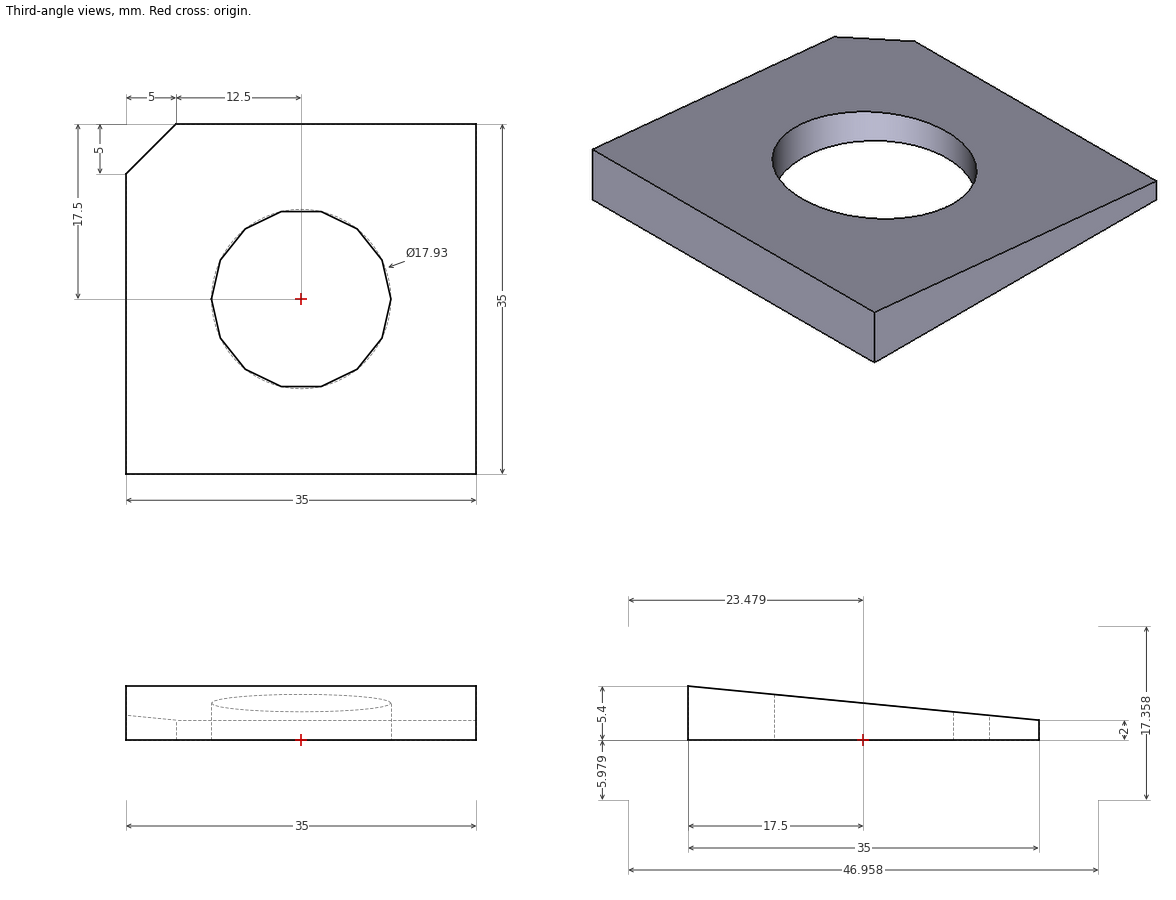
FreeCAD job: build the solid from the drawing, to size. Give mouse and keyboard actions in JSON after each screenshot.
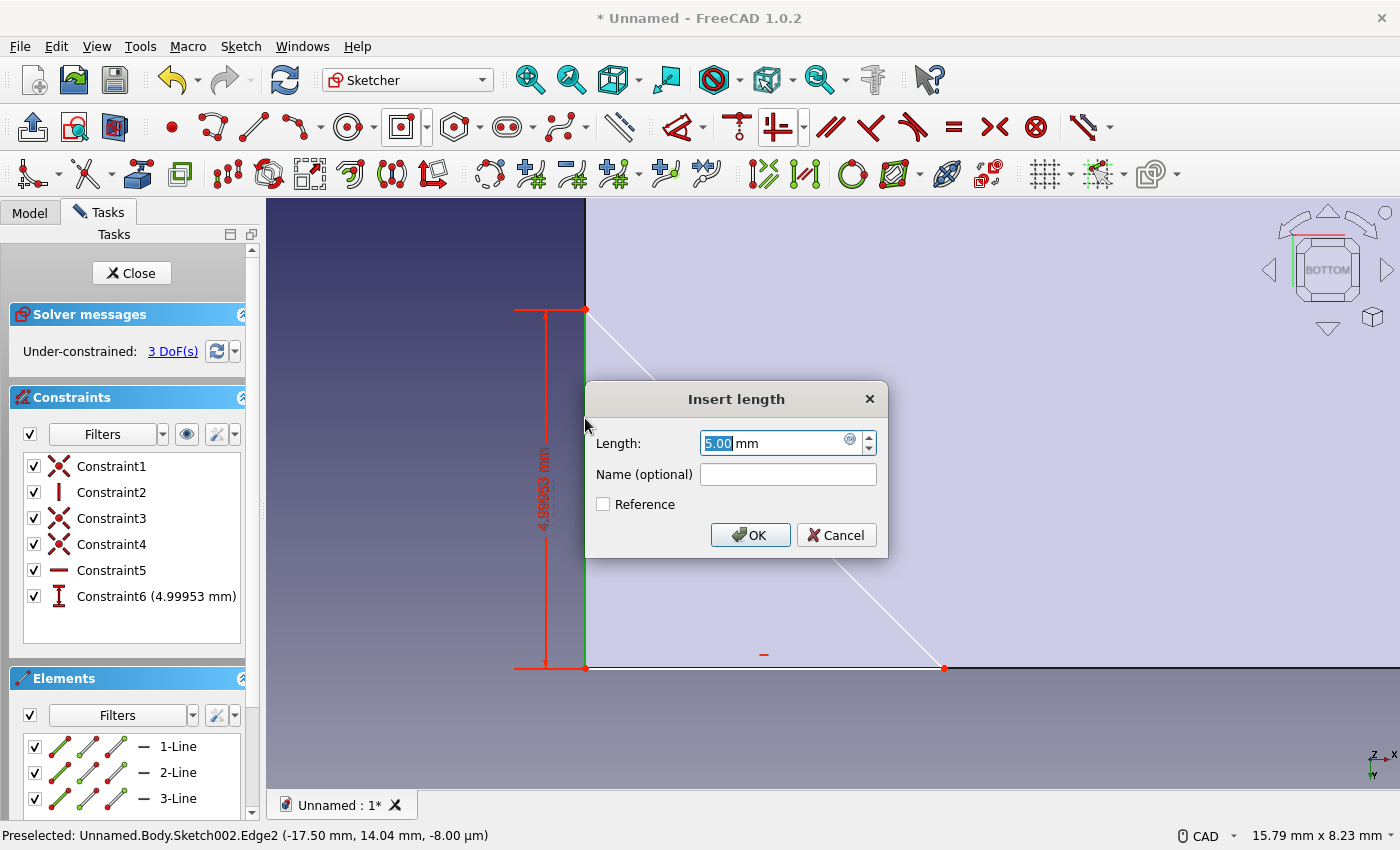
{"action": "type", "text": "5"}
{"action": "key", "text": "Return"}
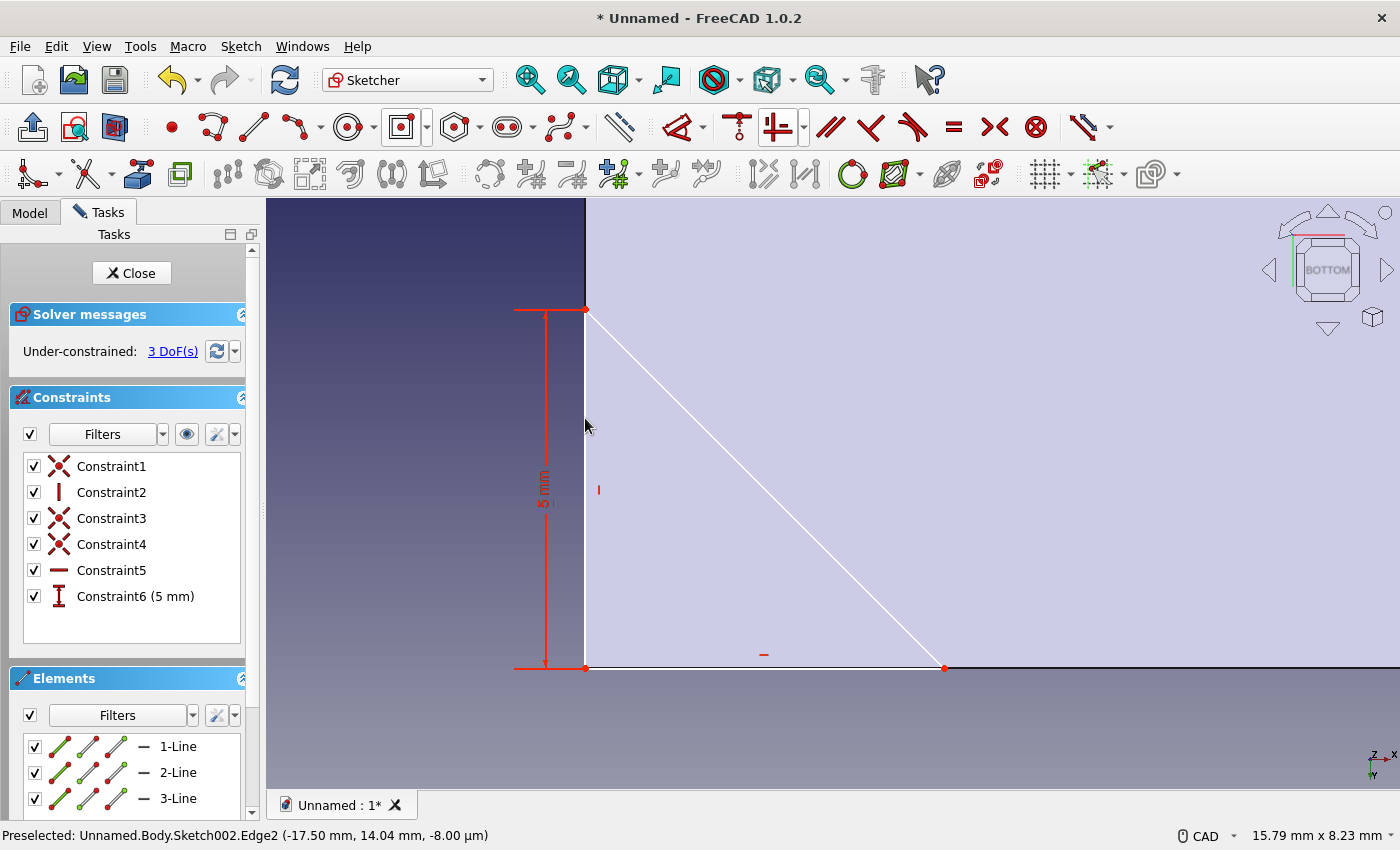
{"action": "left_click", "coordinate": [693, 669]}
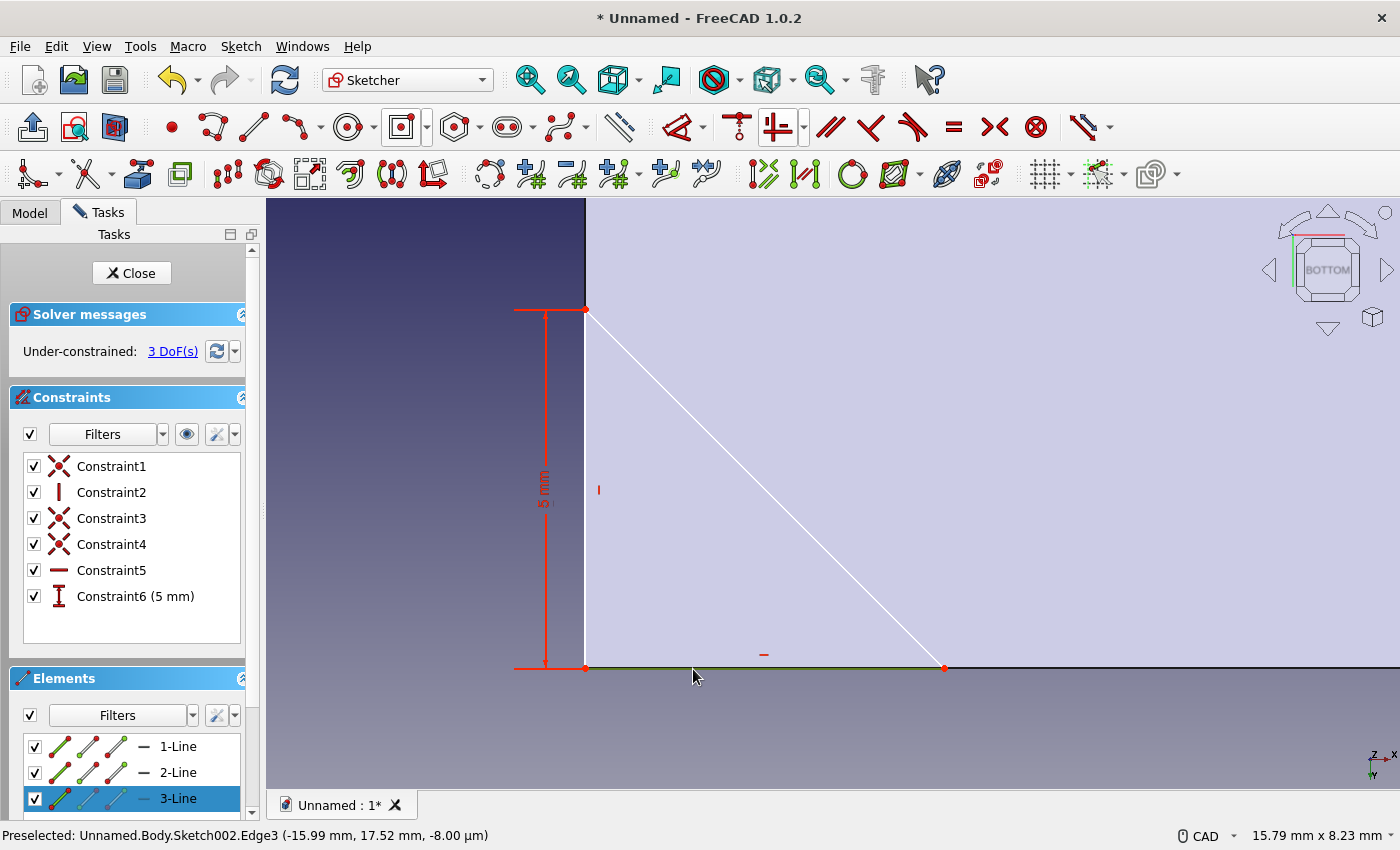
{"action": "key", "text": "l"}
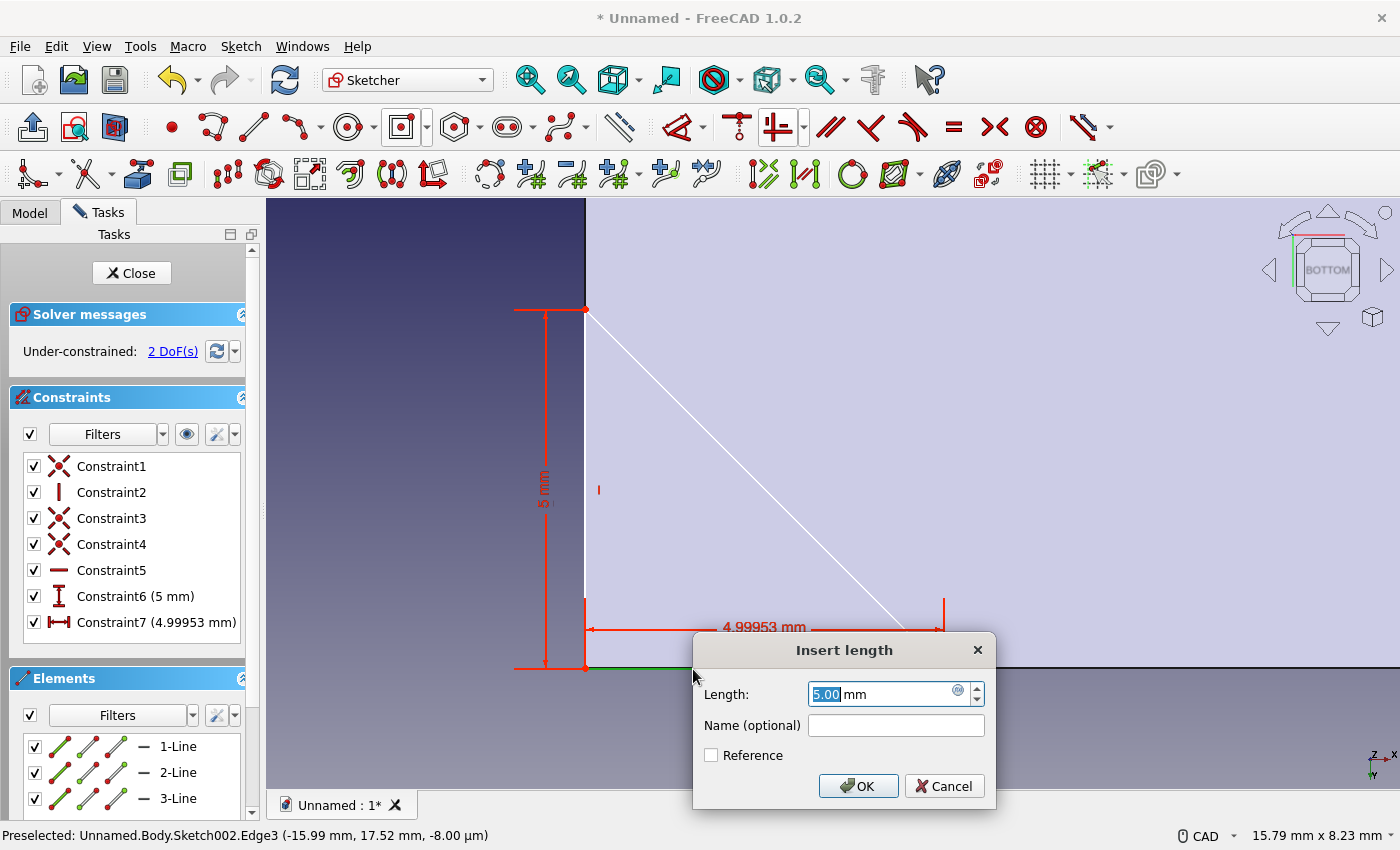
{"action": "type", "text": "5"}
{"action": "key", "text": "Return"}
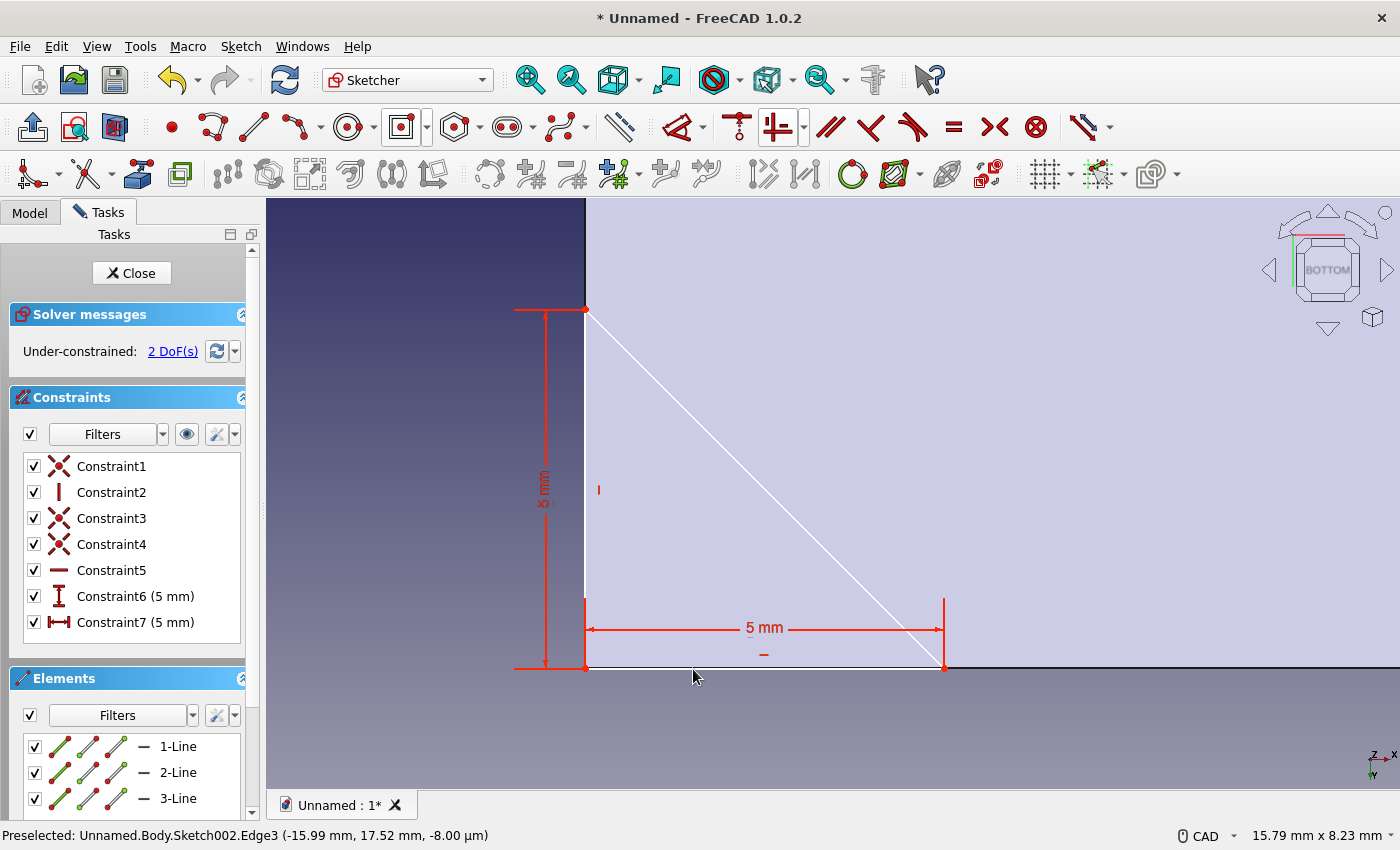
{"action": "left_click", "coordinate": [944, 669]}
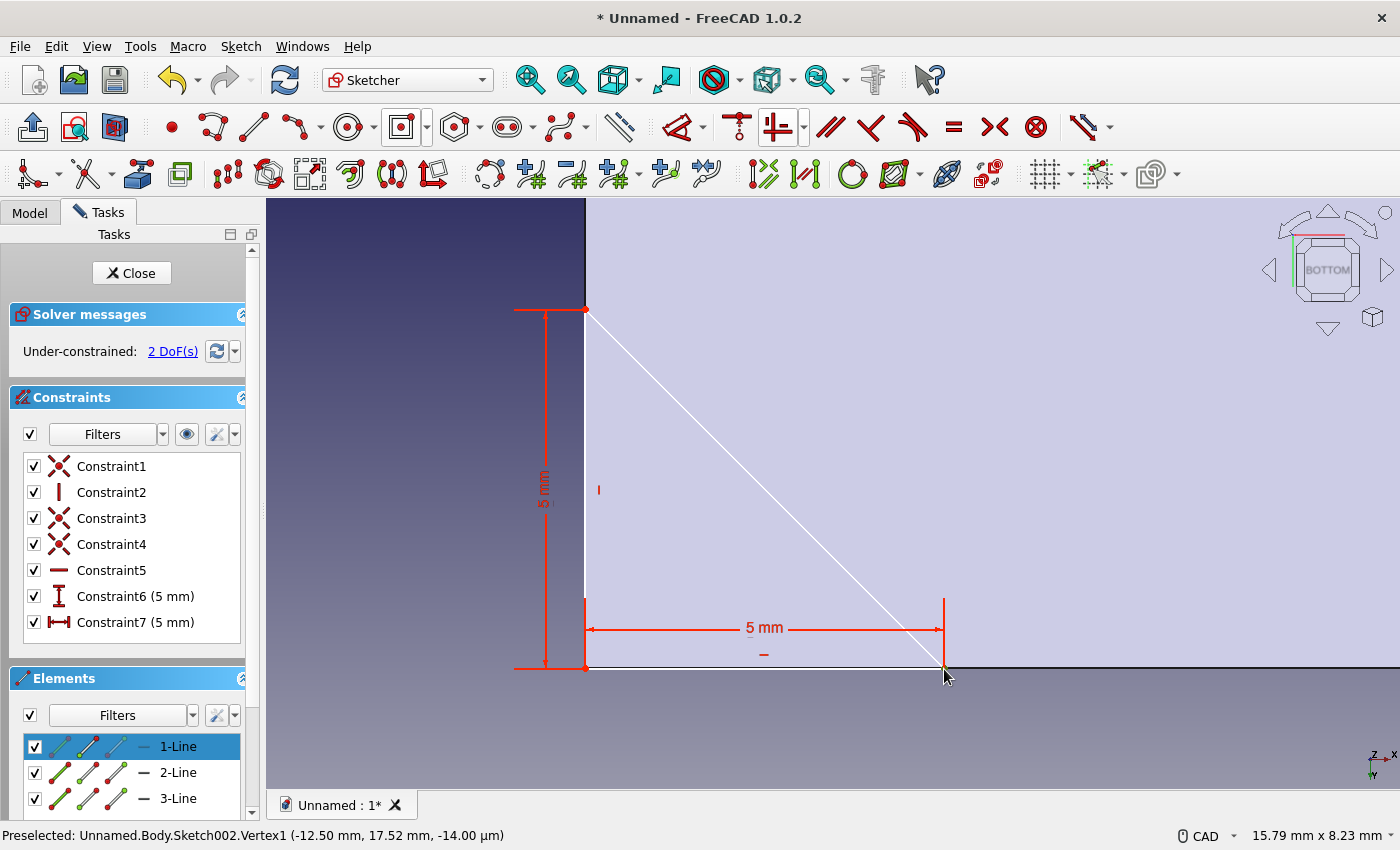
{"action": "key", "text": "l"}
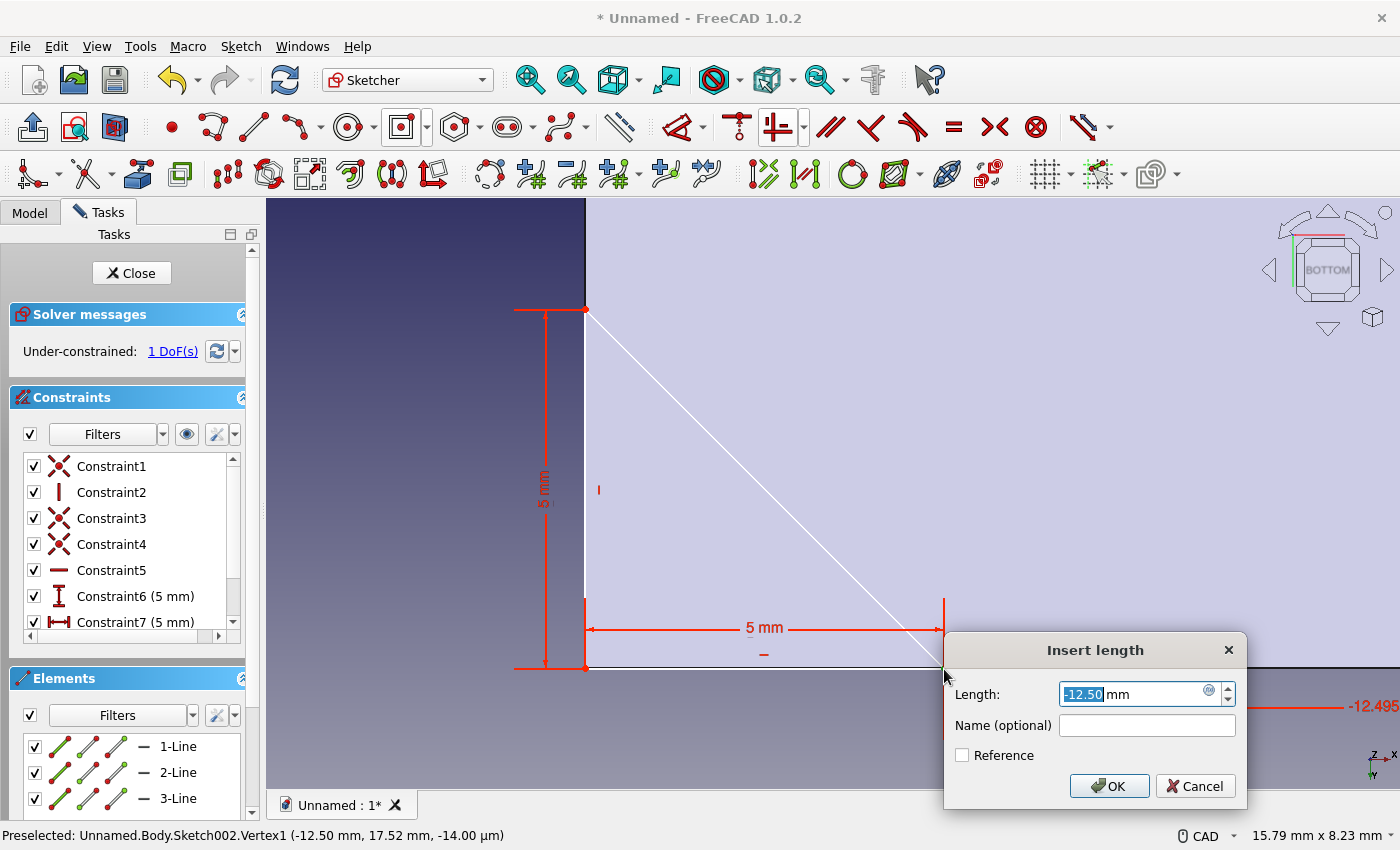
{"action": "type", "text": "-12.5"}
{"action": "key", "text": "Return"}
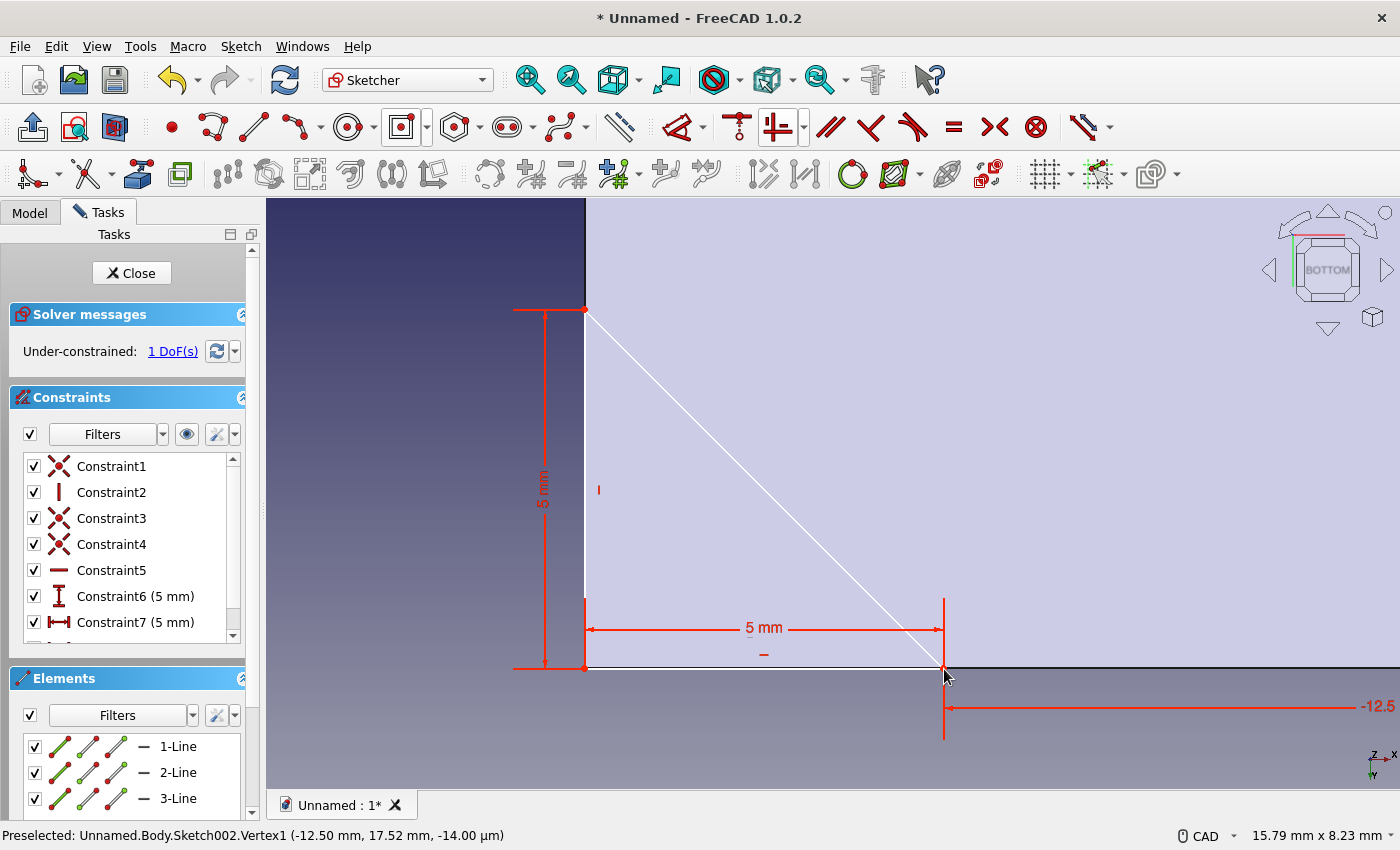
{"action": "left_click", "coordinate": [944, 669]}